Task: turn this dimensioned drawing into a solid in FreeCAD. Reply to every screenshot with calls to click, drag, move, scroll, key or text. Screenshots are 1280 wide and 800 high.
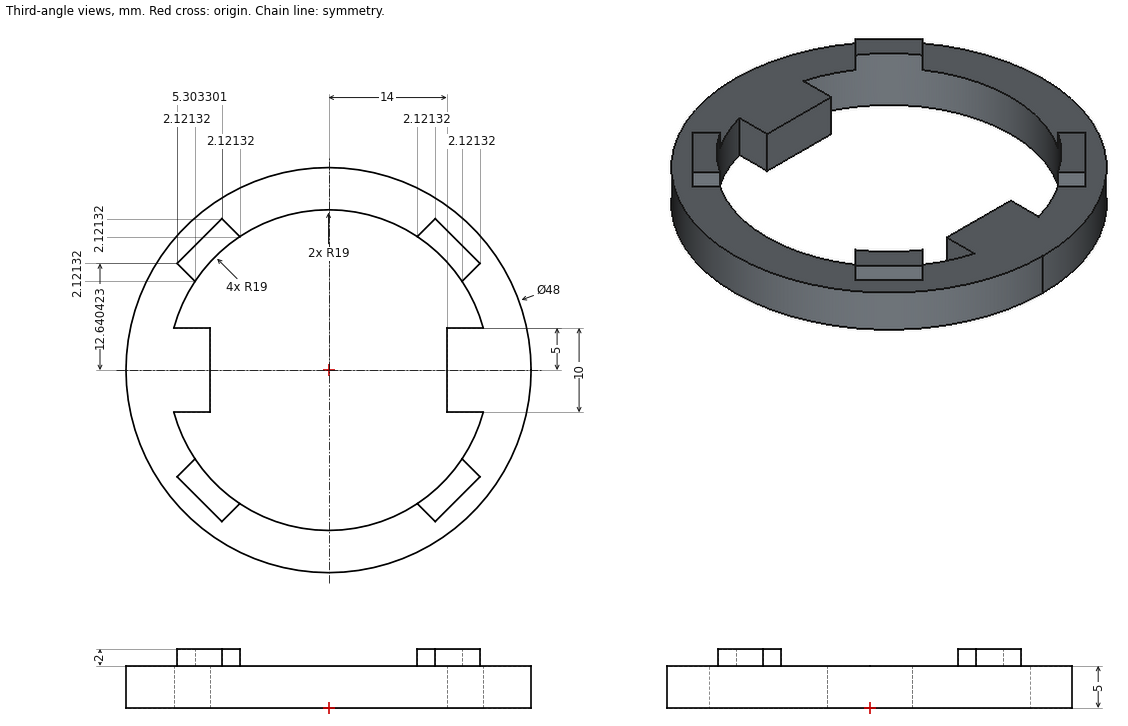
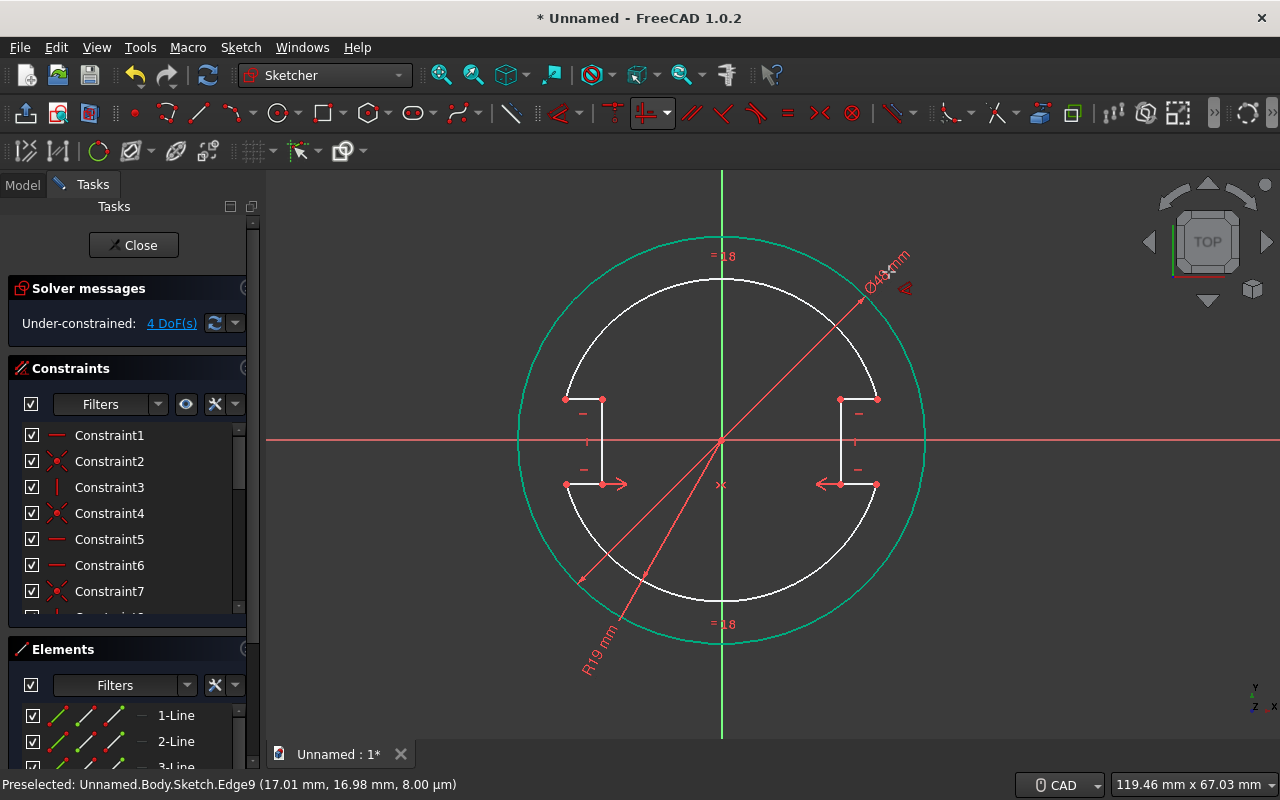
click(841, 425)
click(875, 422)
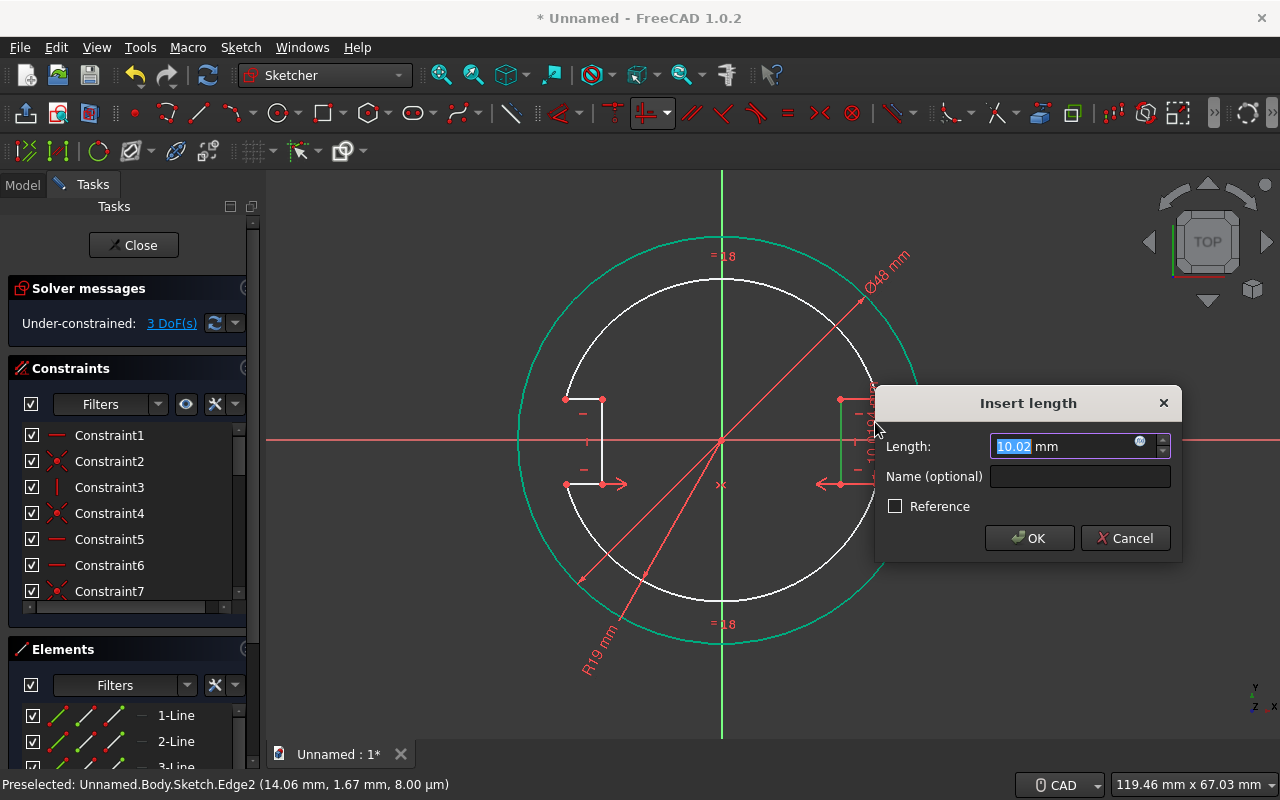
text(10)
key(Return)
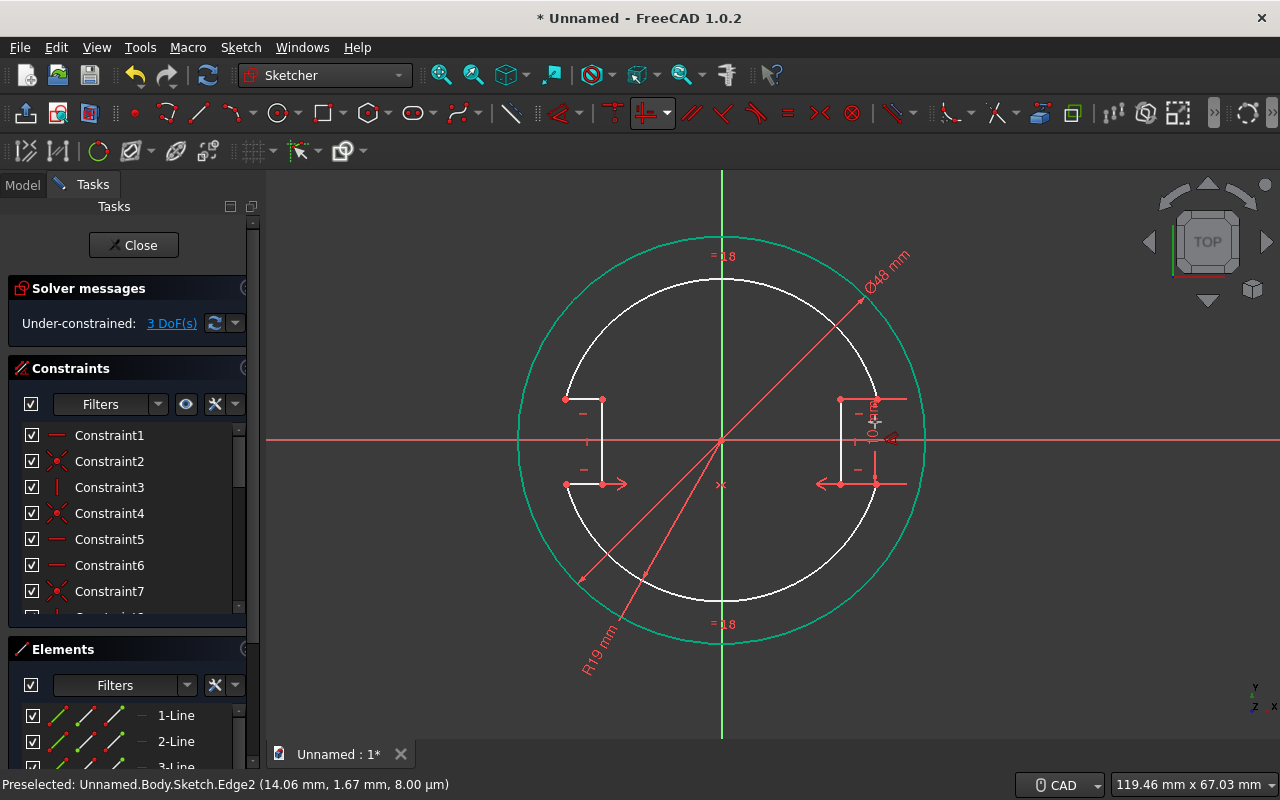
click(602, 459)
click(568, 422)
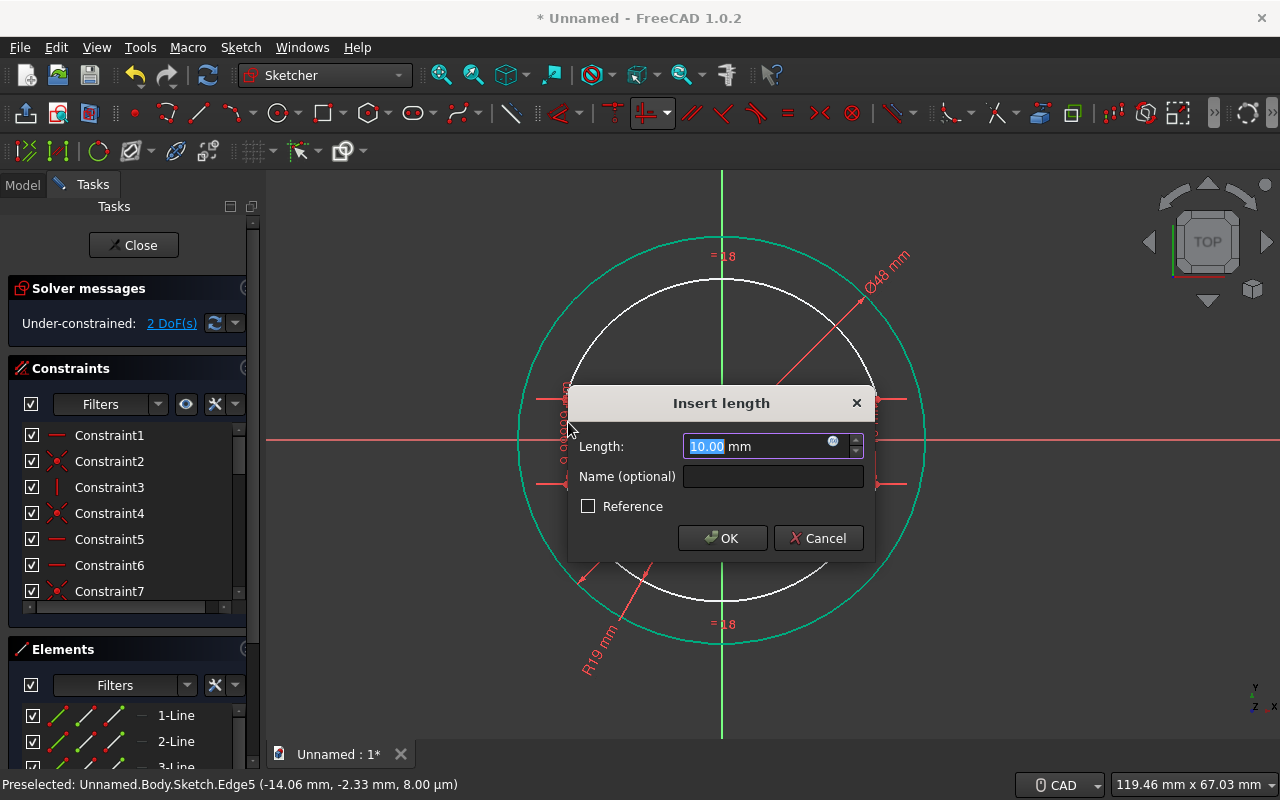
text(10)
key(Return)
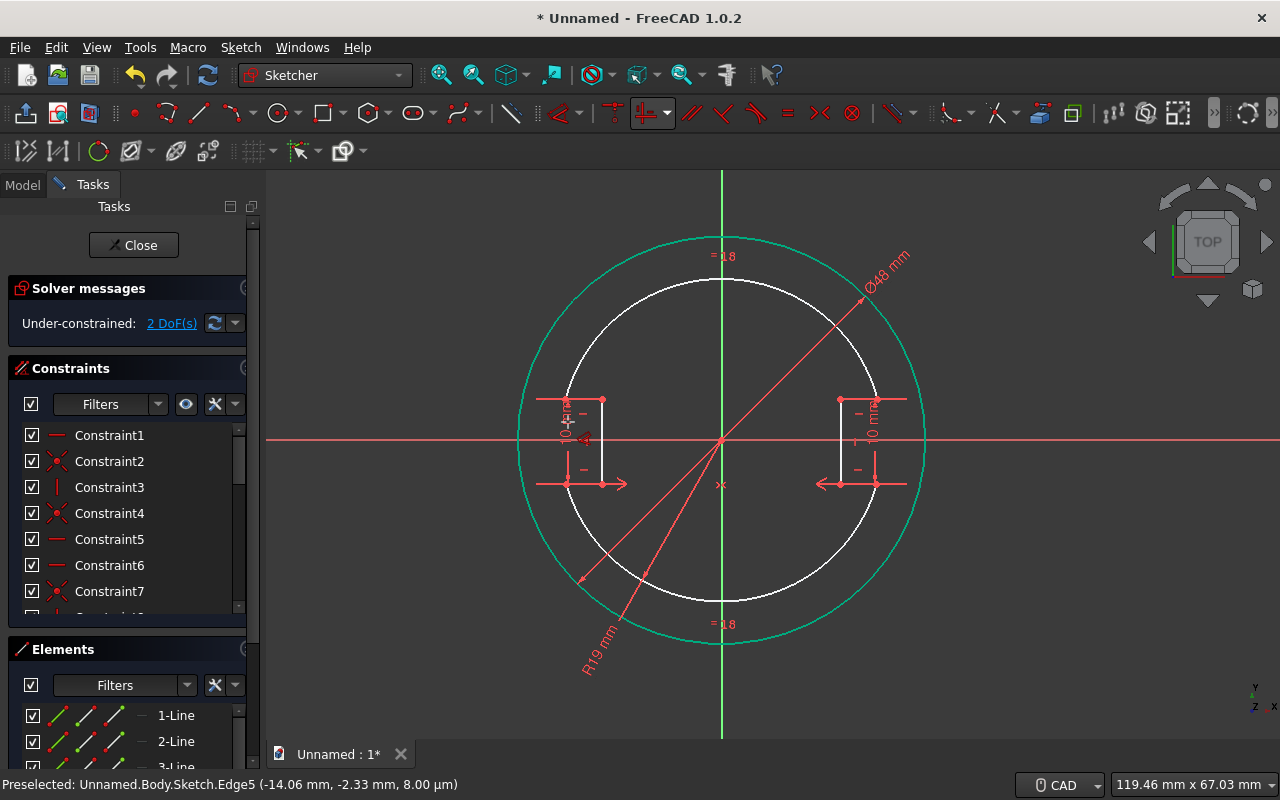
click(878, 399)
click(688, 420)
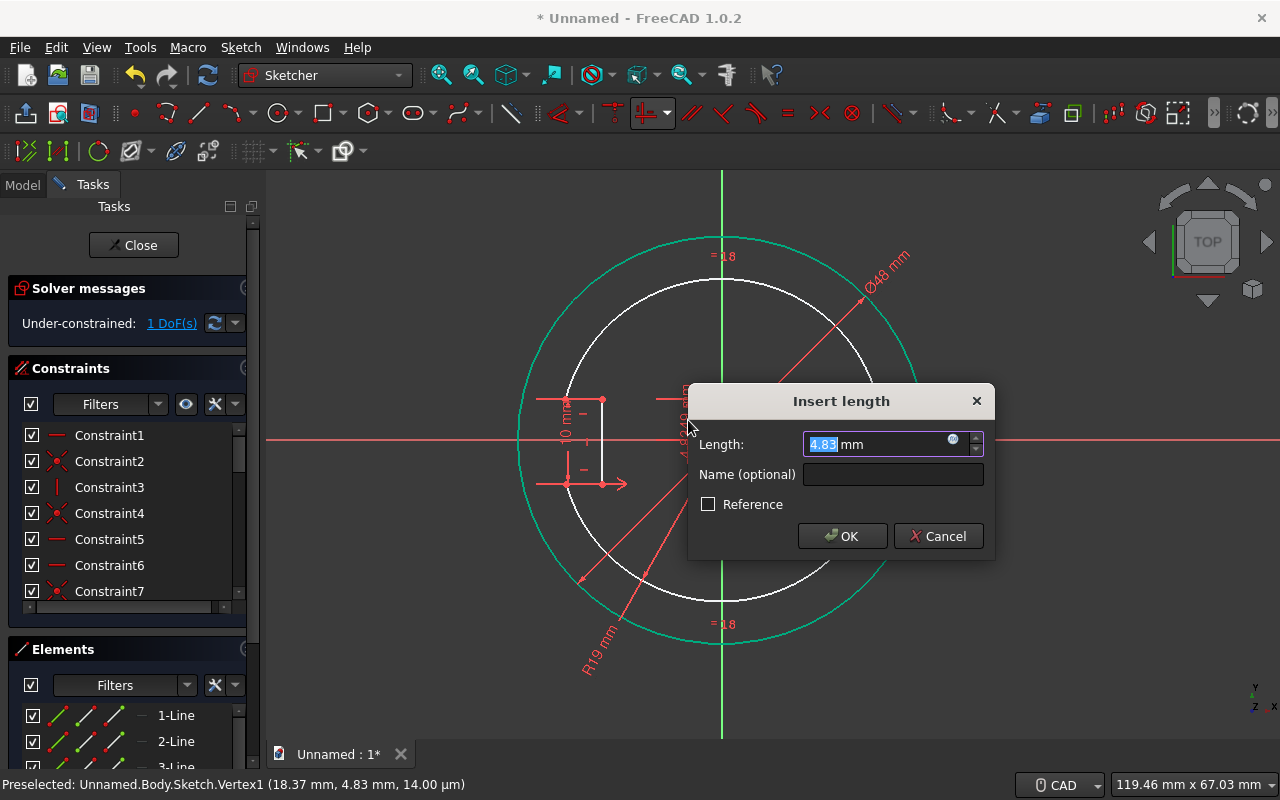
text(5)
key(Return)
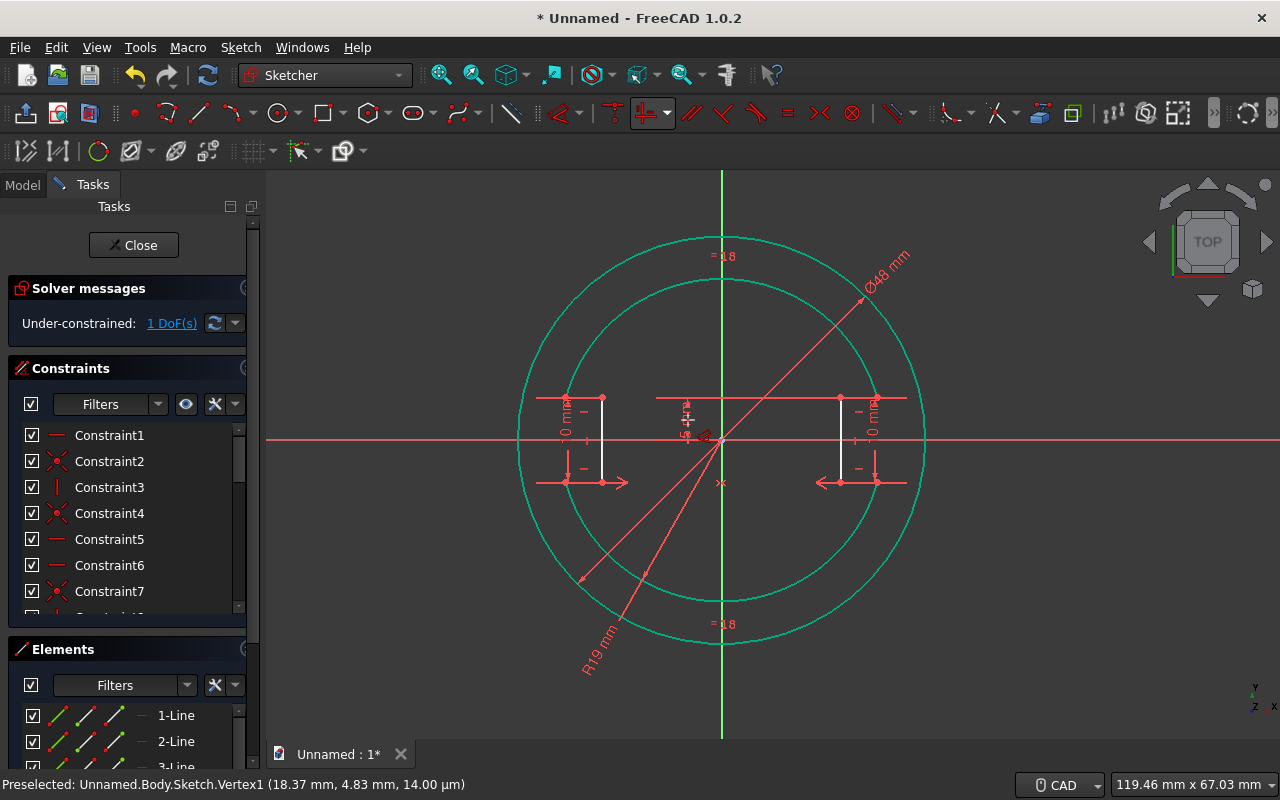
click(841, 398)
click(781, 364)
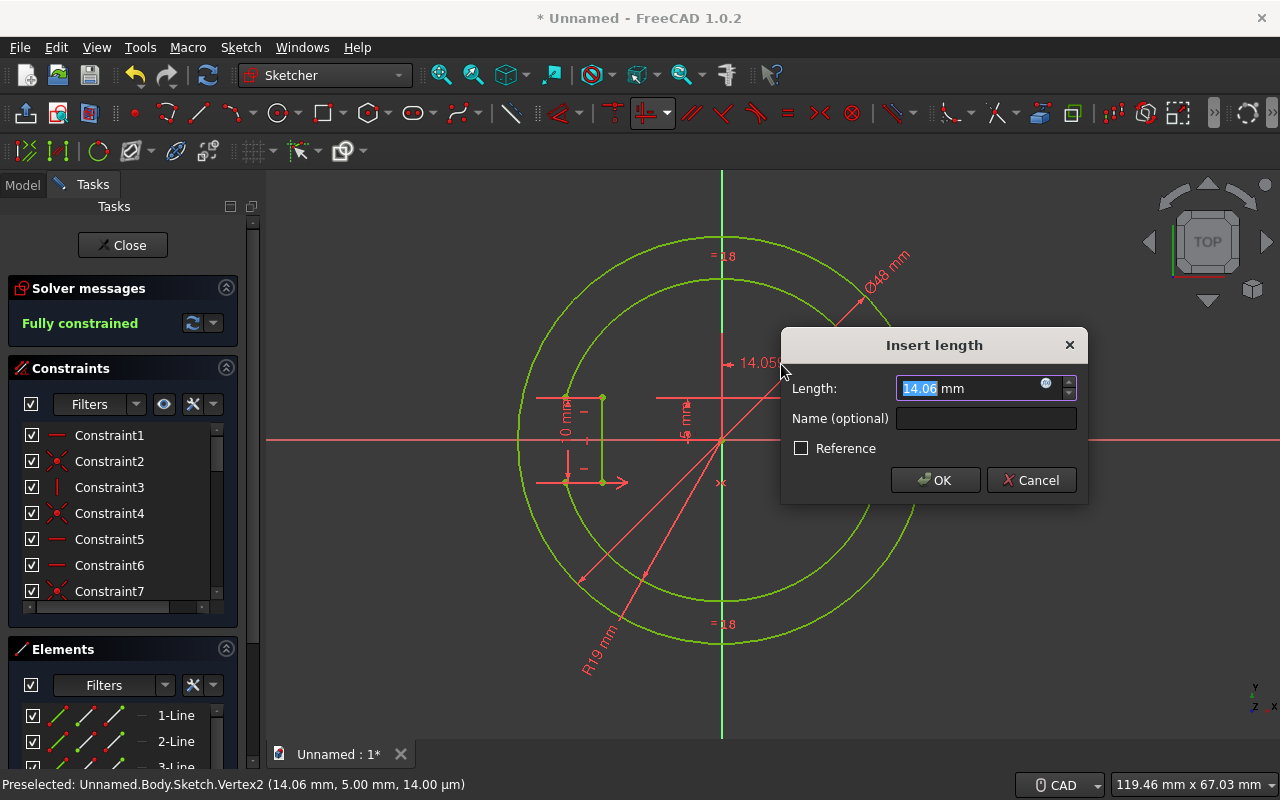
text(14)
key(Return)
key(Escape)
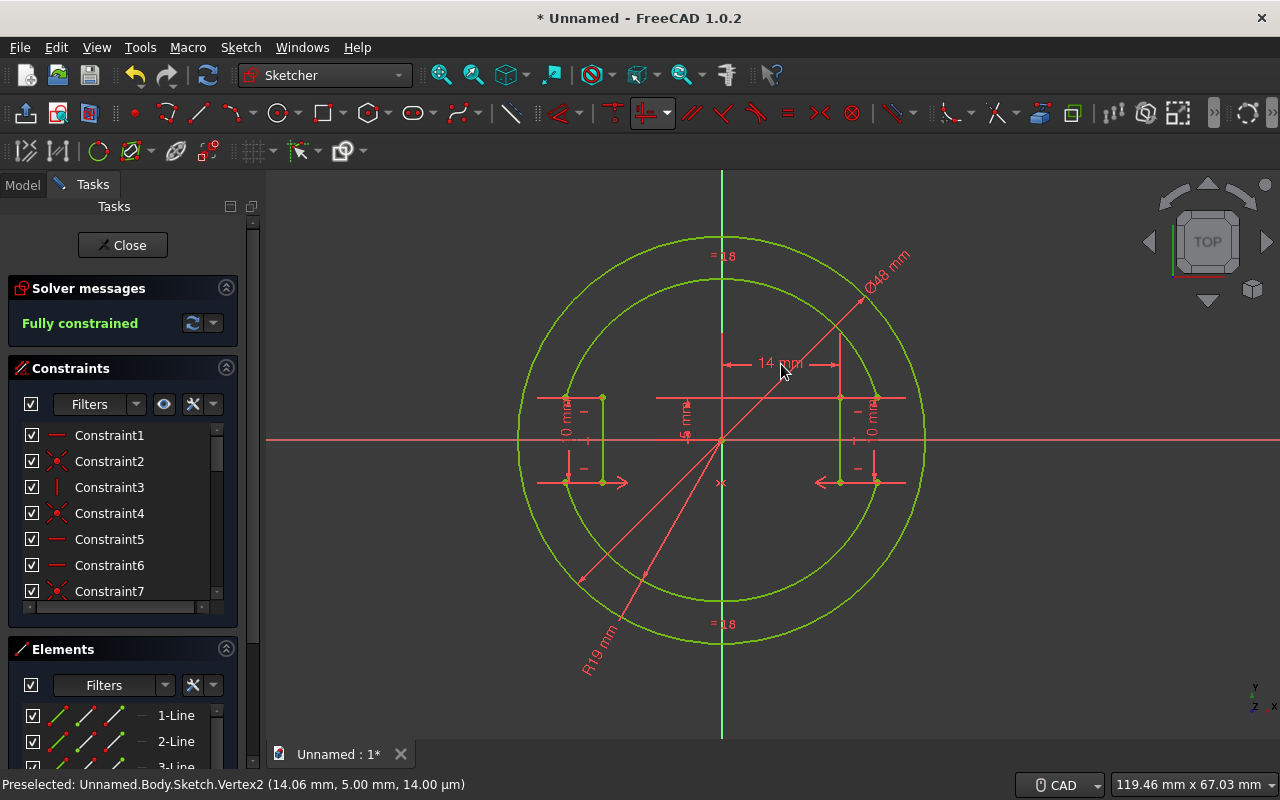
click(123, 245)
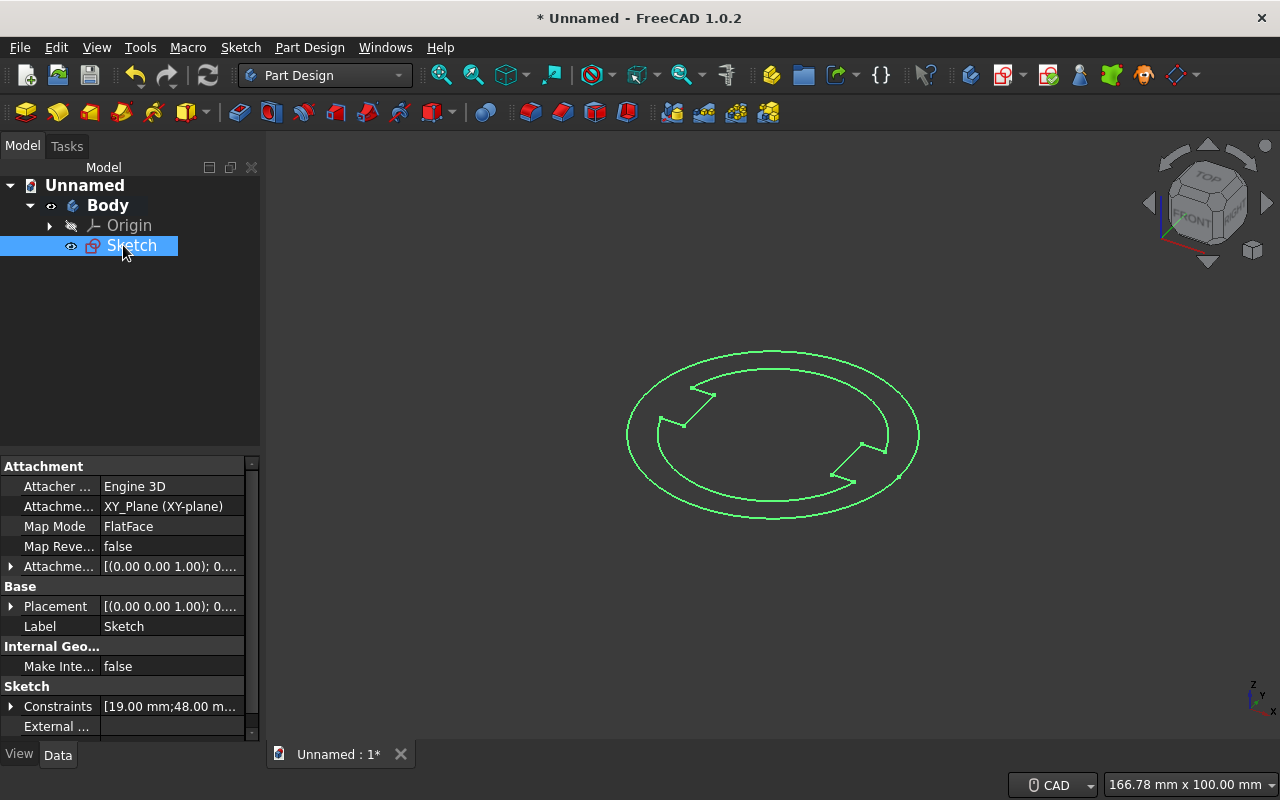
click(26, 112)